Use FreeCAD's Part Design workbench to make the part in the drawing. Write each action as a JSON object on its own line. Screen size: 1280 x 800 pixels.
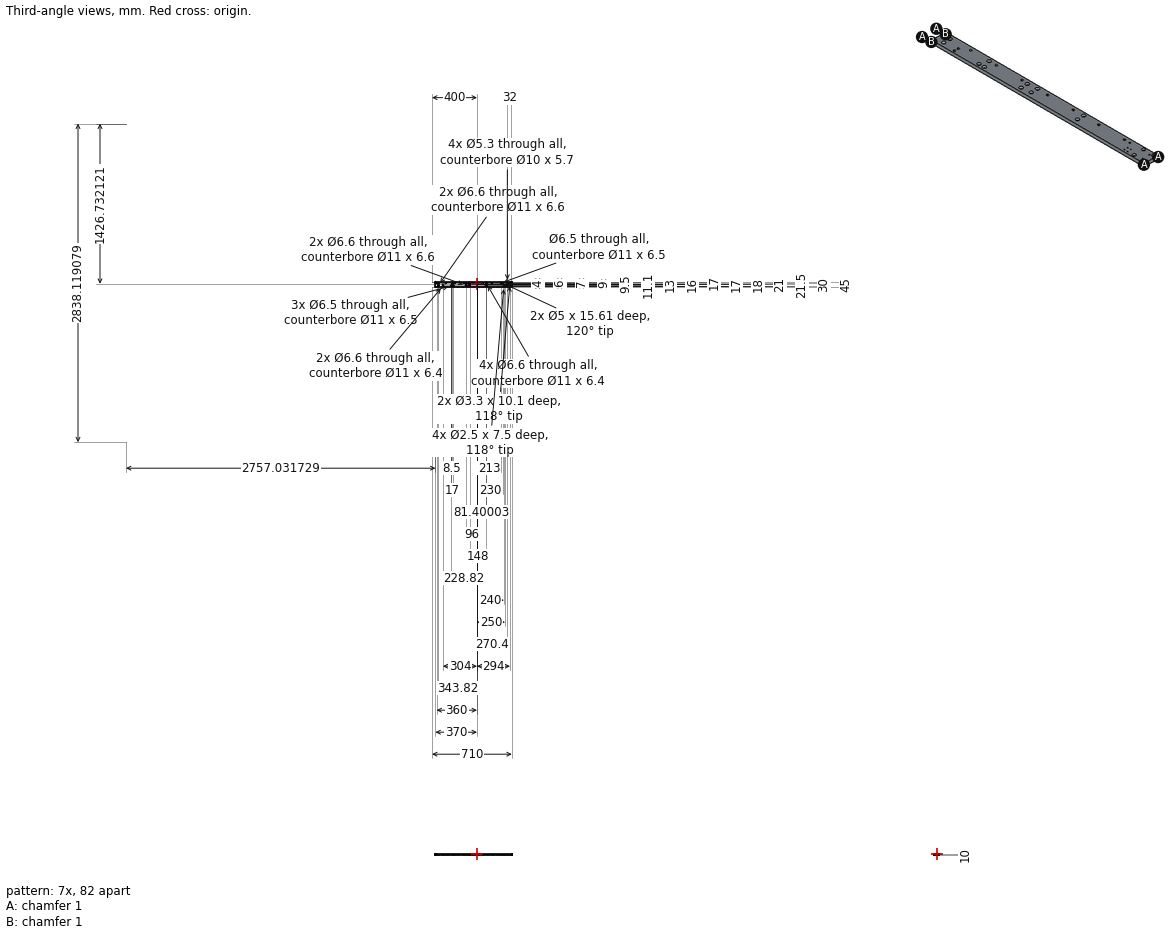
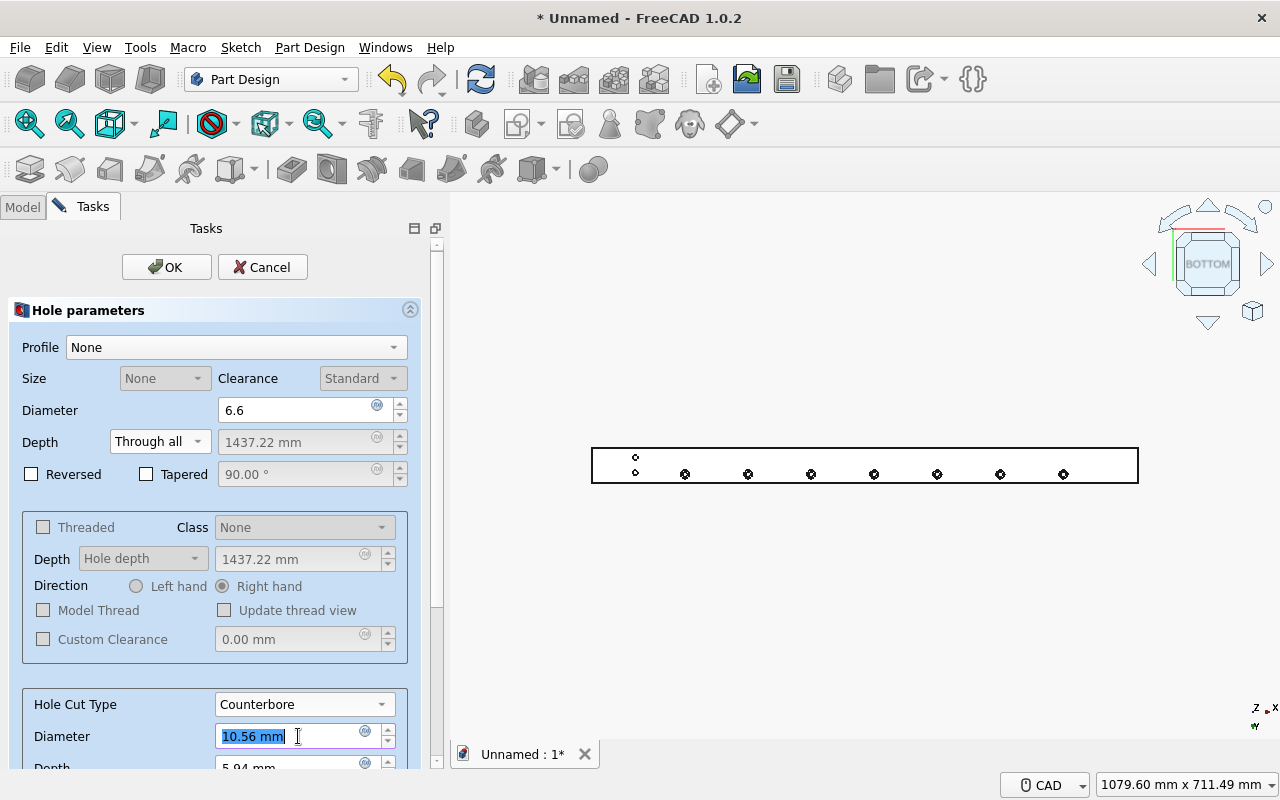
{"action": "type", "text": "11"}
{"action": "key", "text": "Tab"}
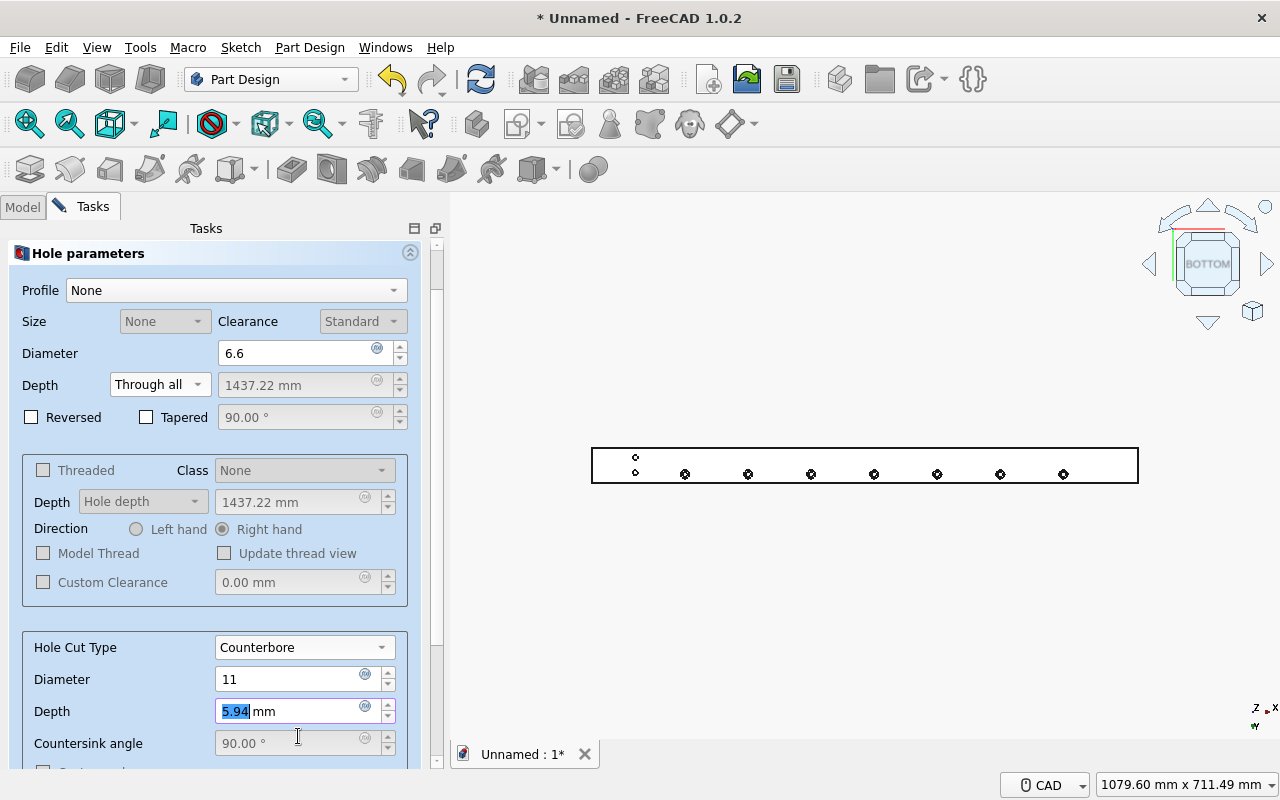
{"action": "type", "text": "6.6"}
{"action": "key", "text": "Tab"}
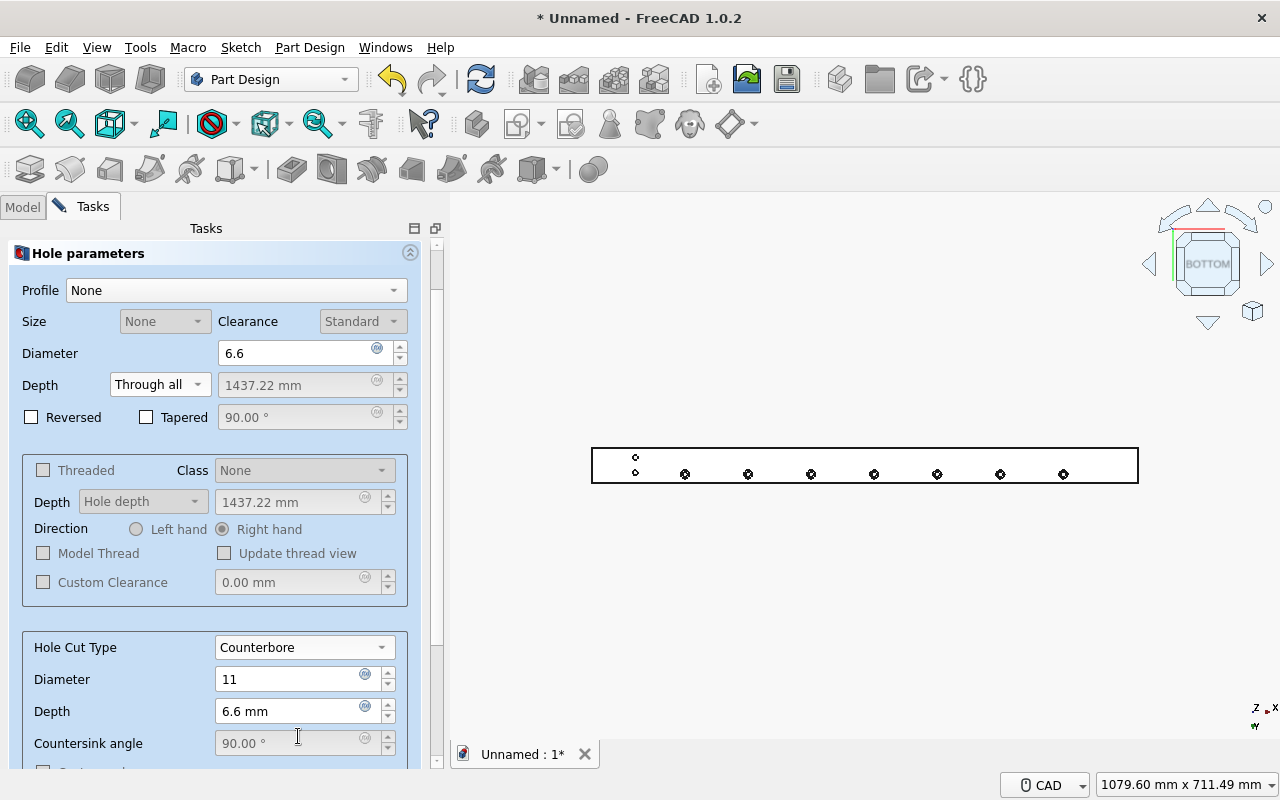
{"action": "scroll", "coordinate": [437, 503], "scroll_direction": "up", "scroll_amount": 2}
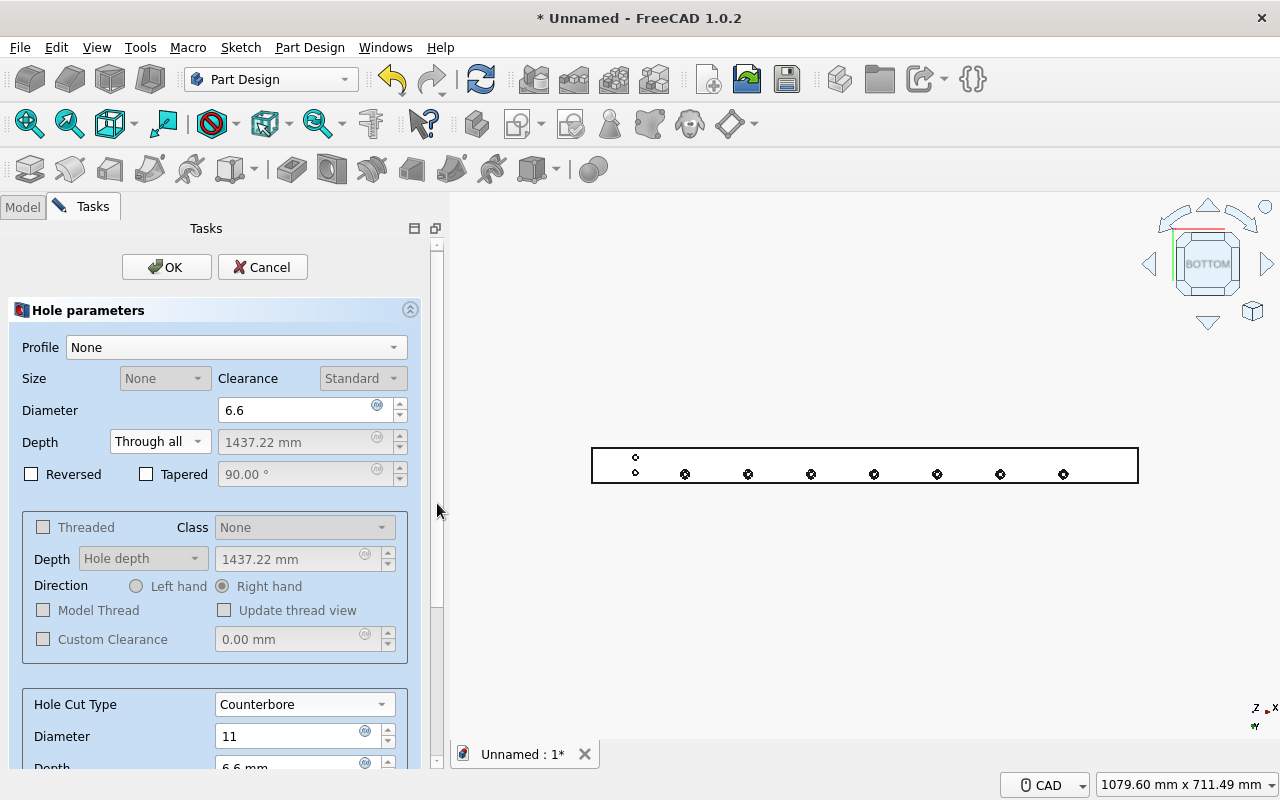
{"action": "left_click", "coordinate": [167, 267]}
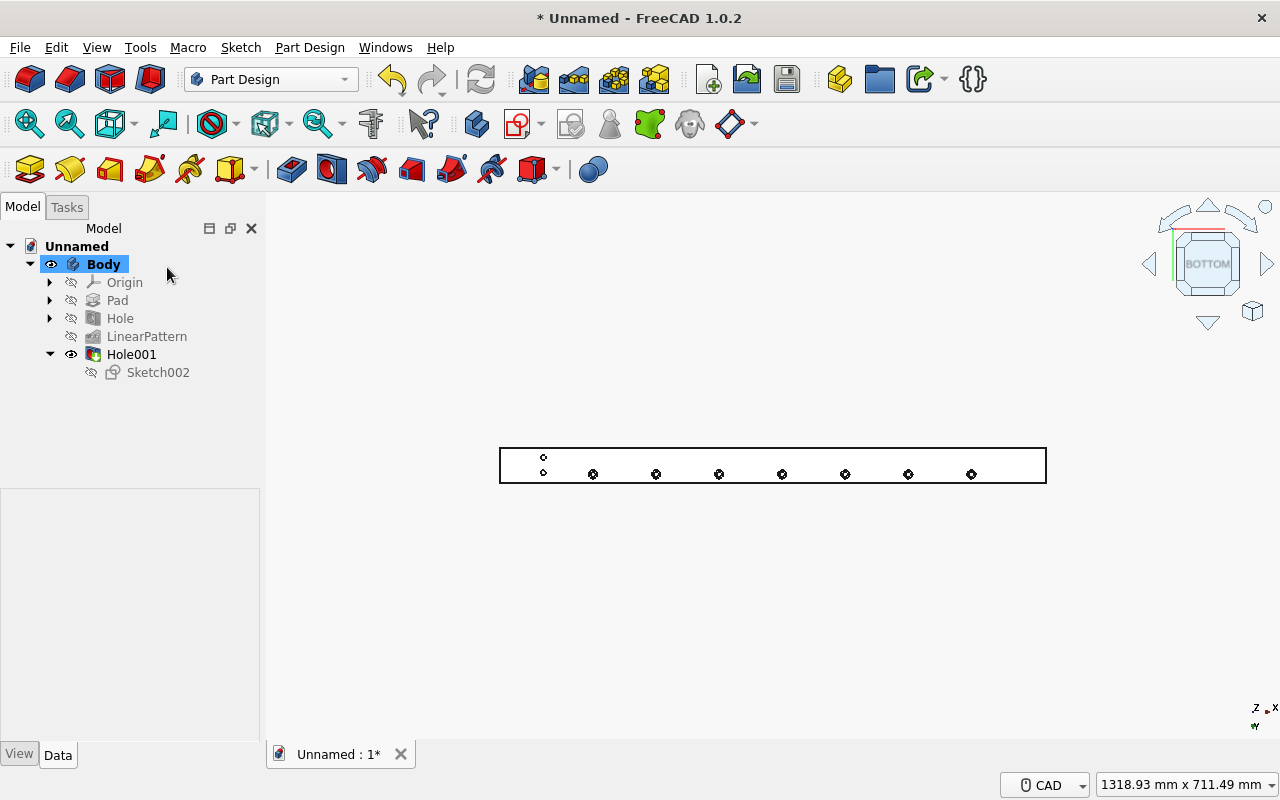
{"action": "key", "text": "0"}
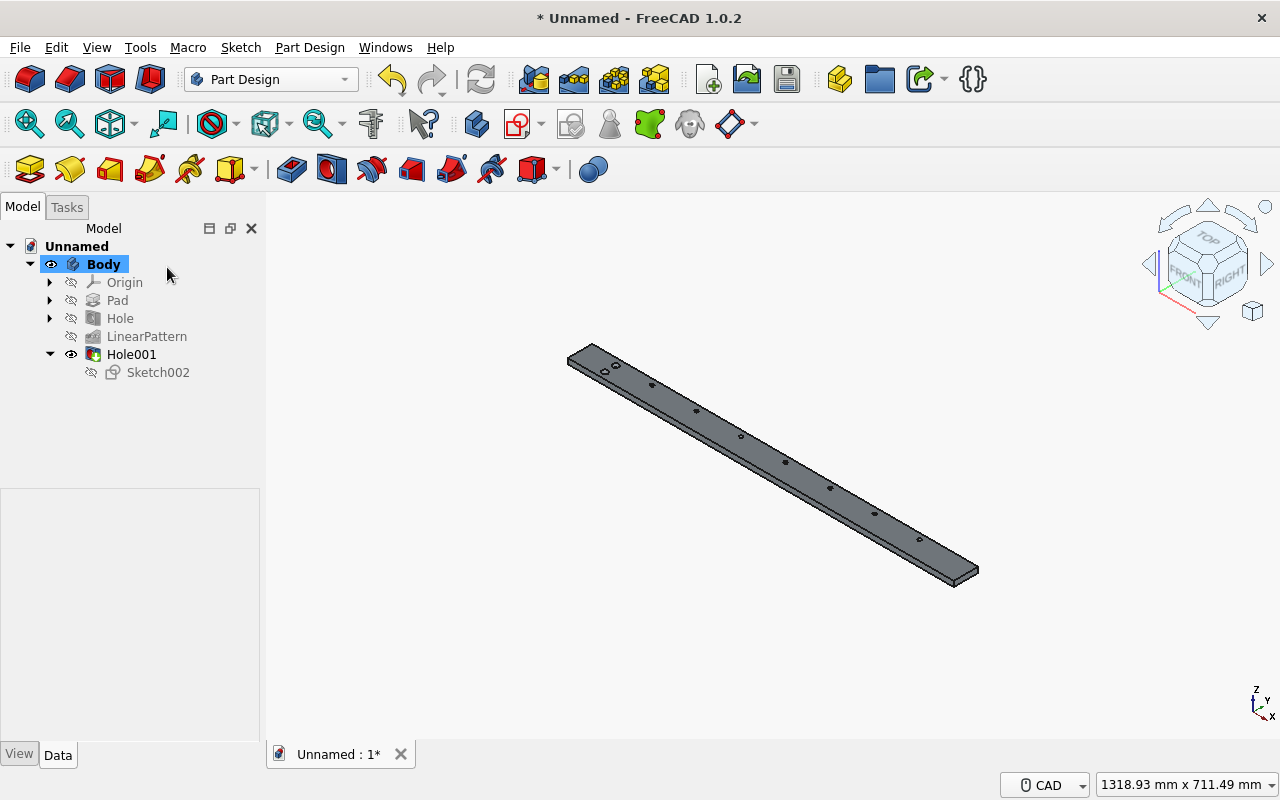
{"action": "left_click", "coordinate": [30, 124]}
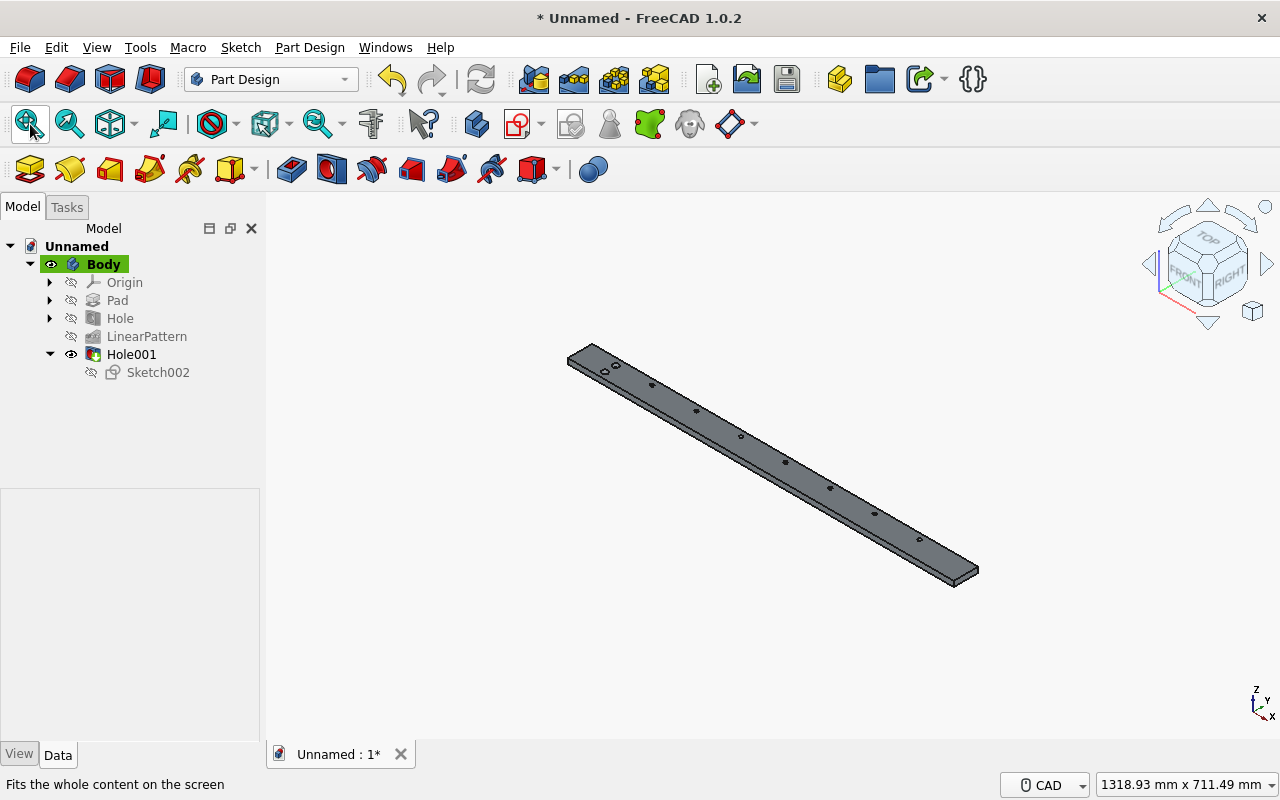
{"action": "left_click", "coordinate": [938, 557]}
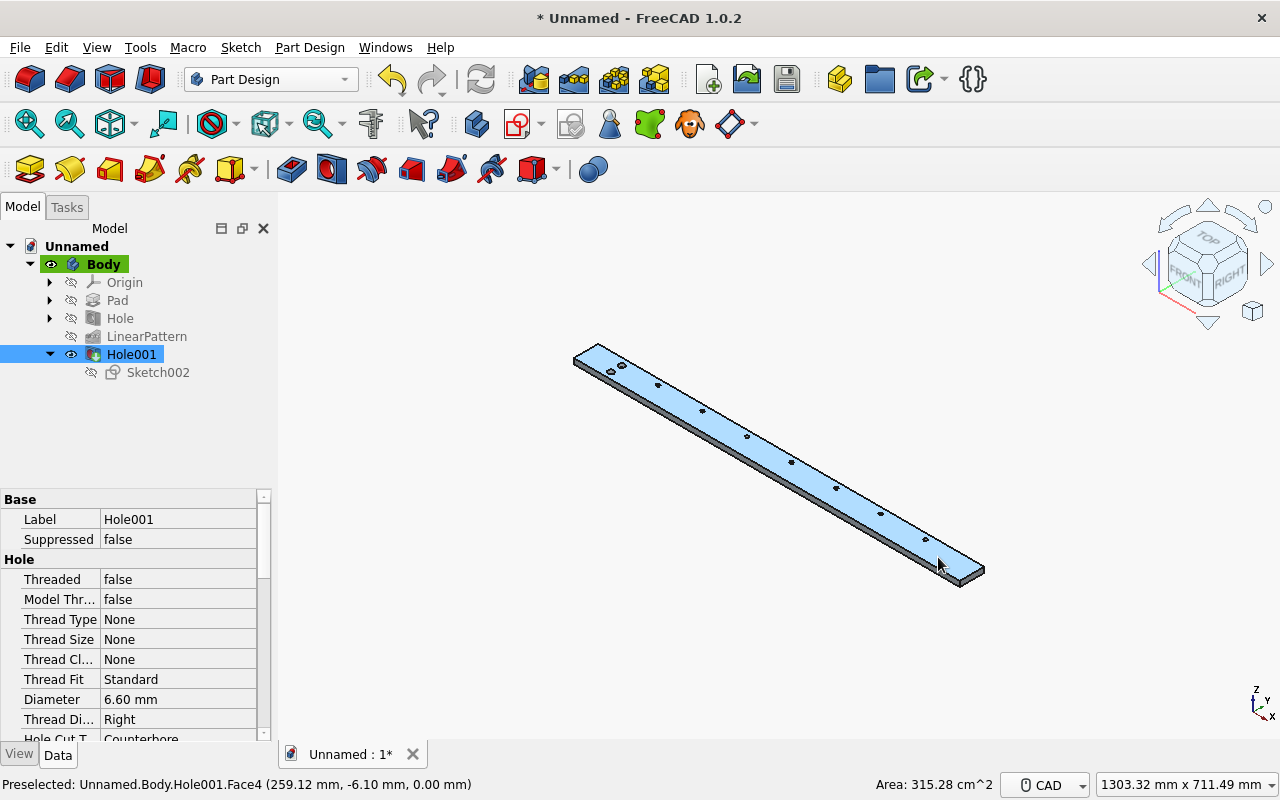
{"action": "left_click", "coordinate": [518, 124]}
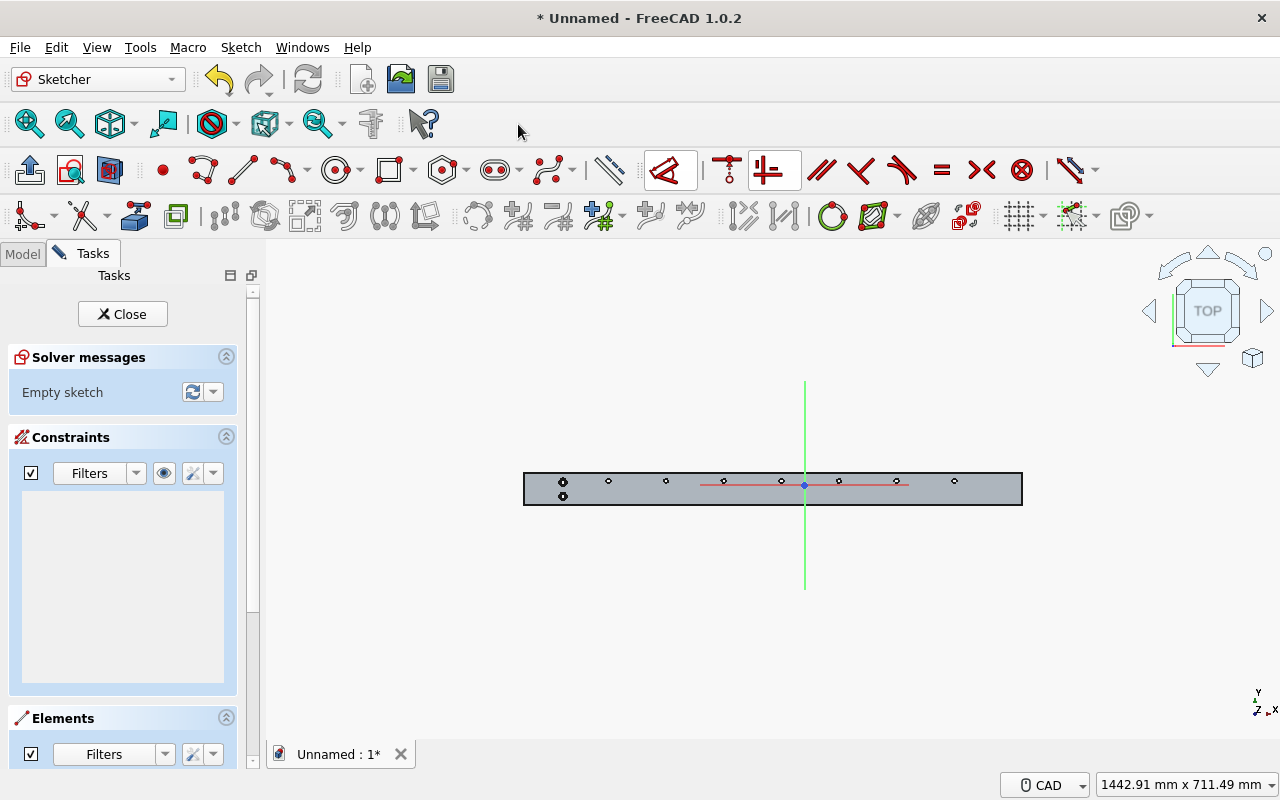
{"action": "scroll", "coordinate": [739, 489], "scroll_direction": "up", "scroll_amount": 14}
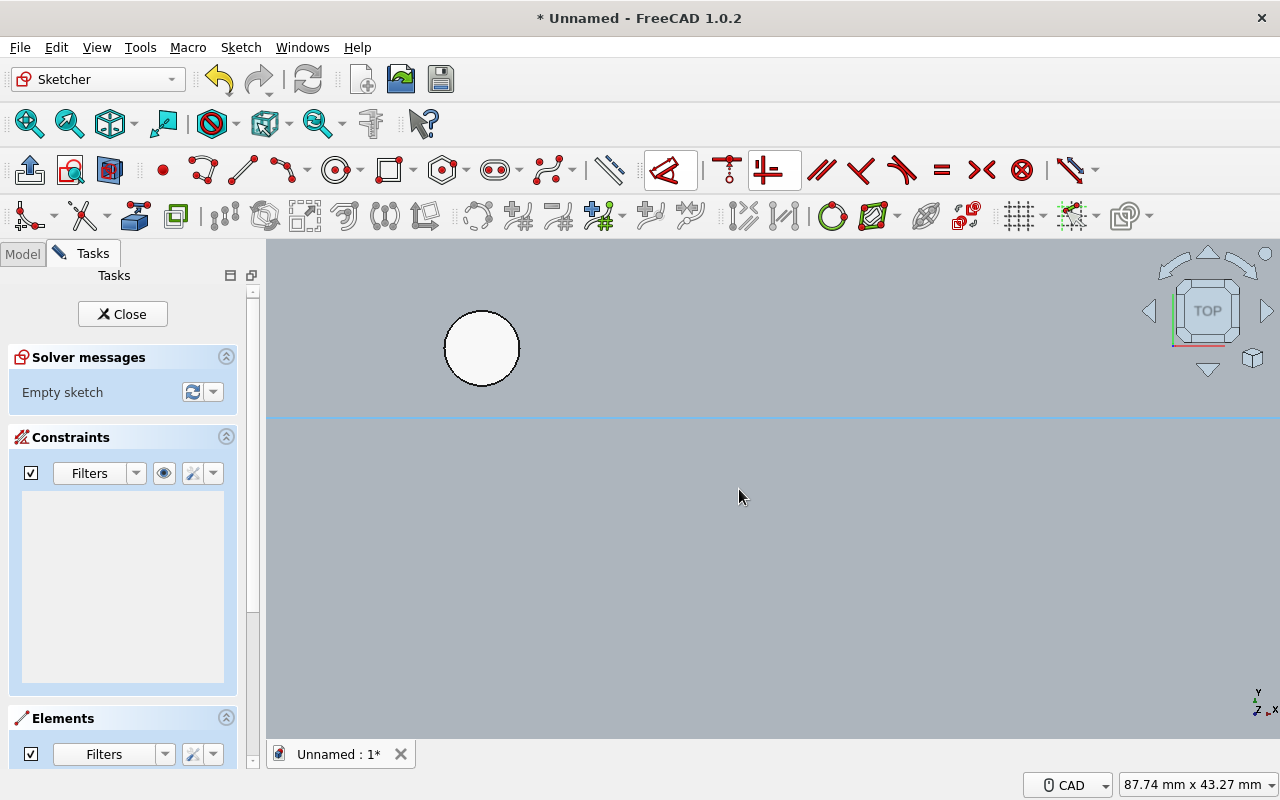
{"action": "left_click", "coordinate": [336, 170]}